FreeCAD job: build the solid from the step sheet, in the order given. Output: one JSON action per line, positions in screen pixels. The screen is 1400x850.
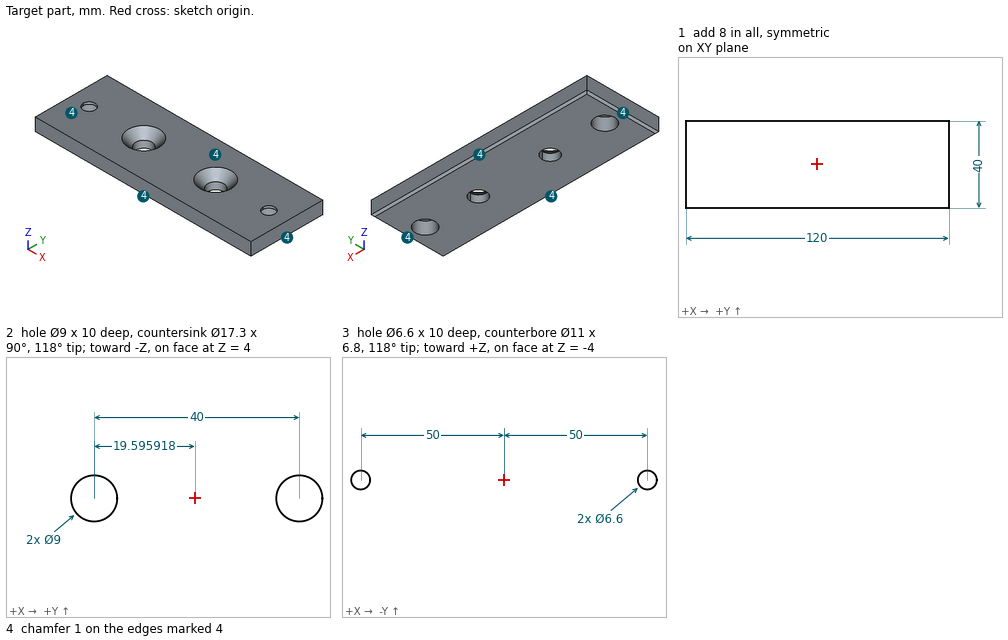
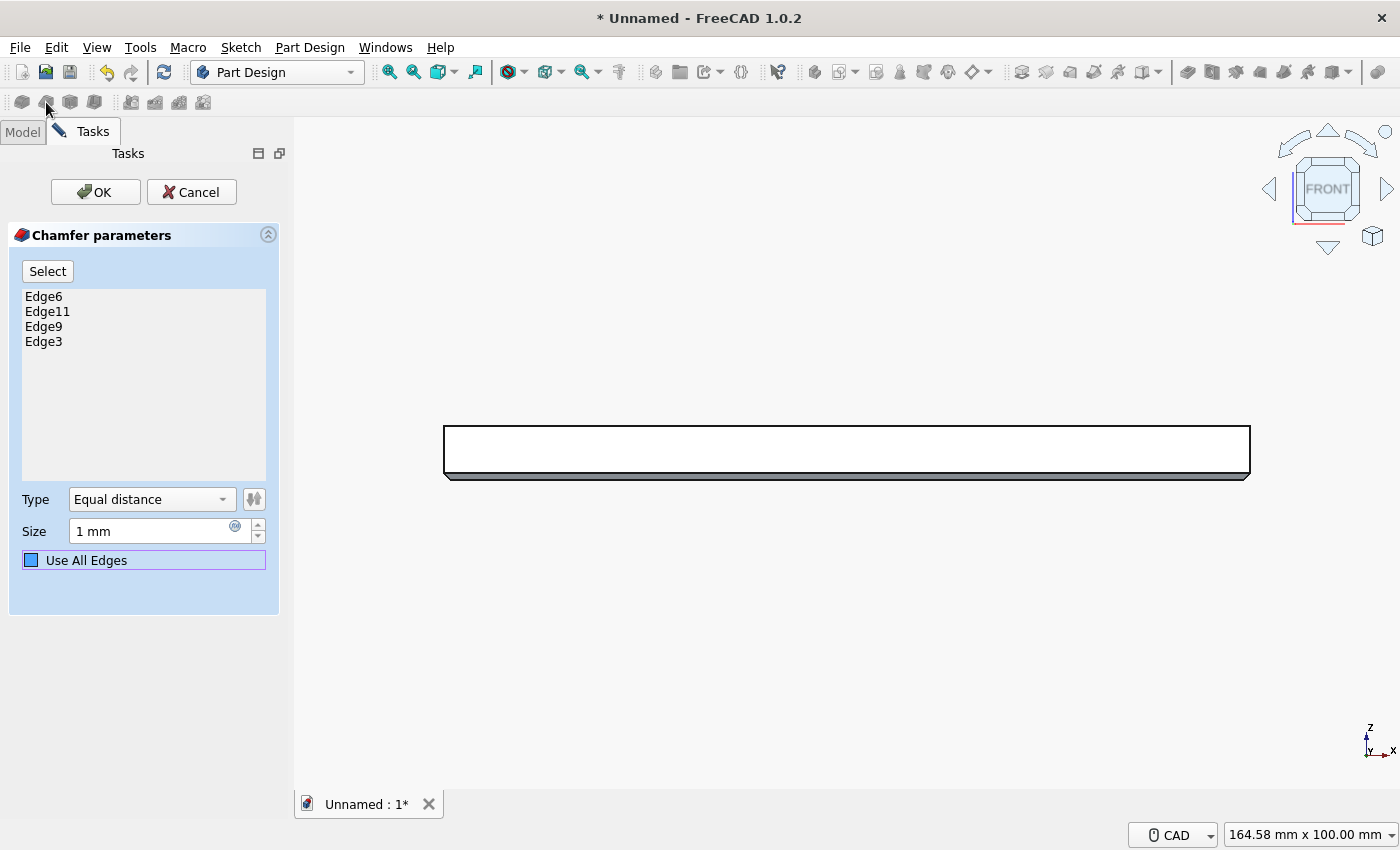
{"action": "left_click", "coordinate": [96, 192]}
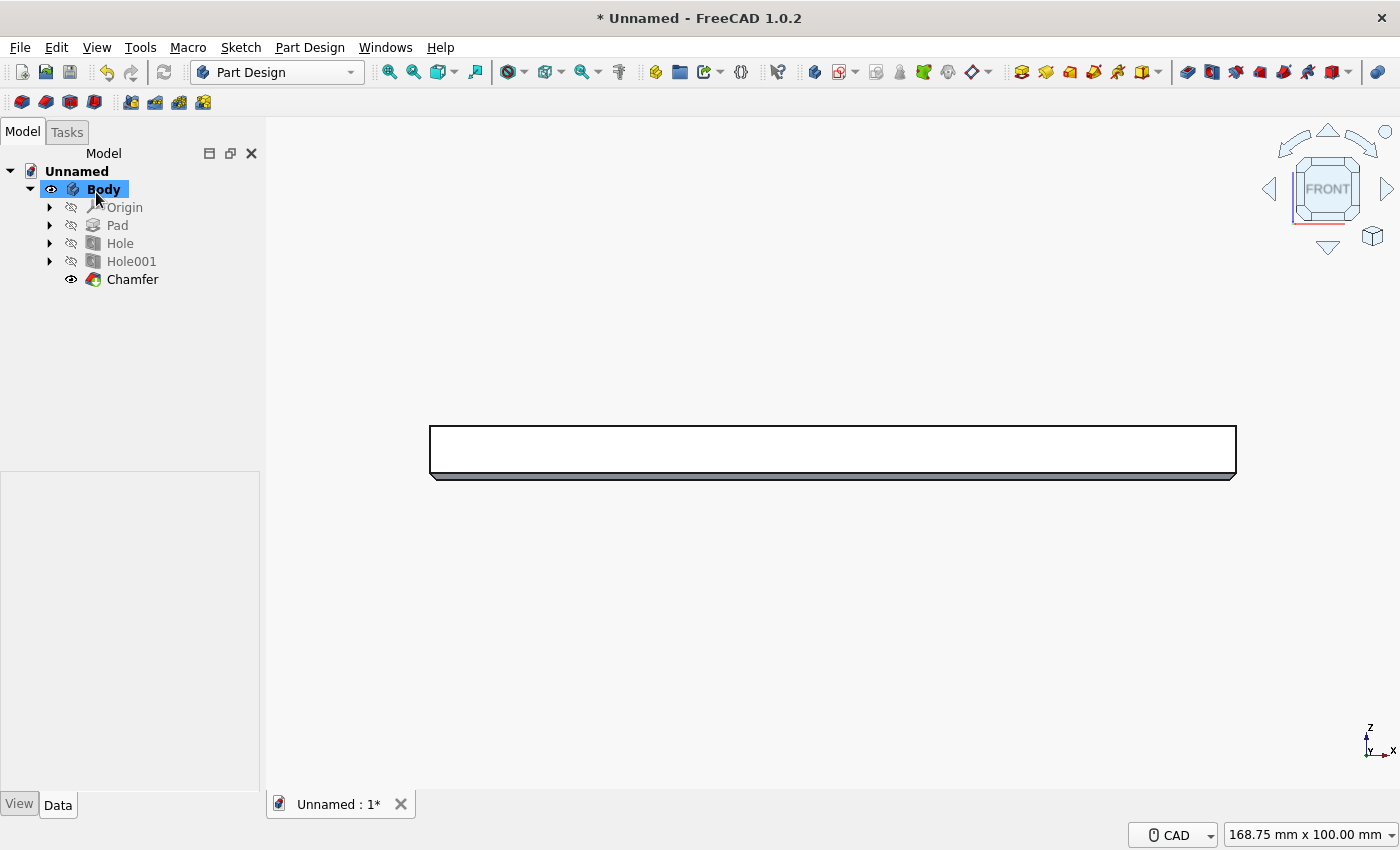
{"action": "key", "text": "0"}